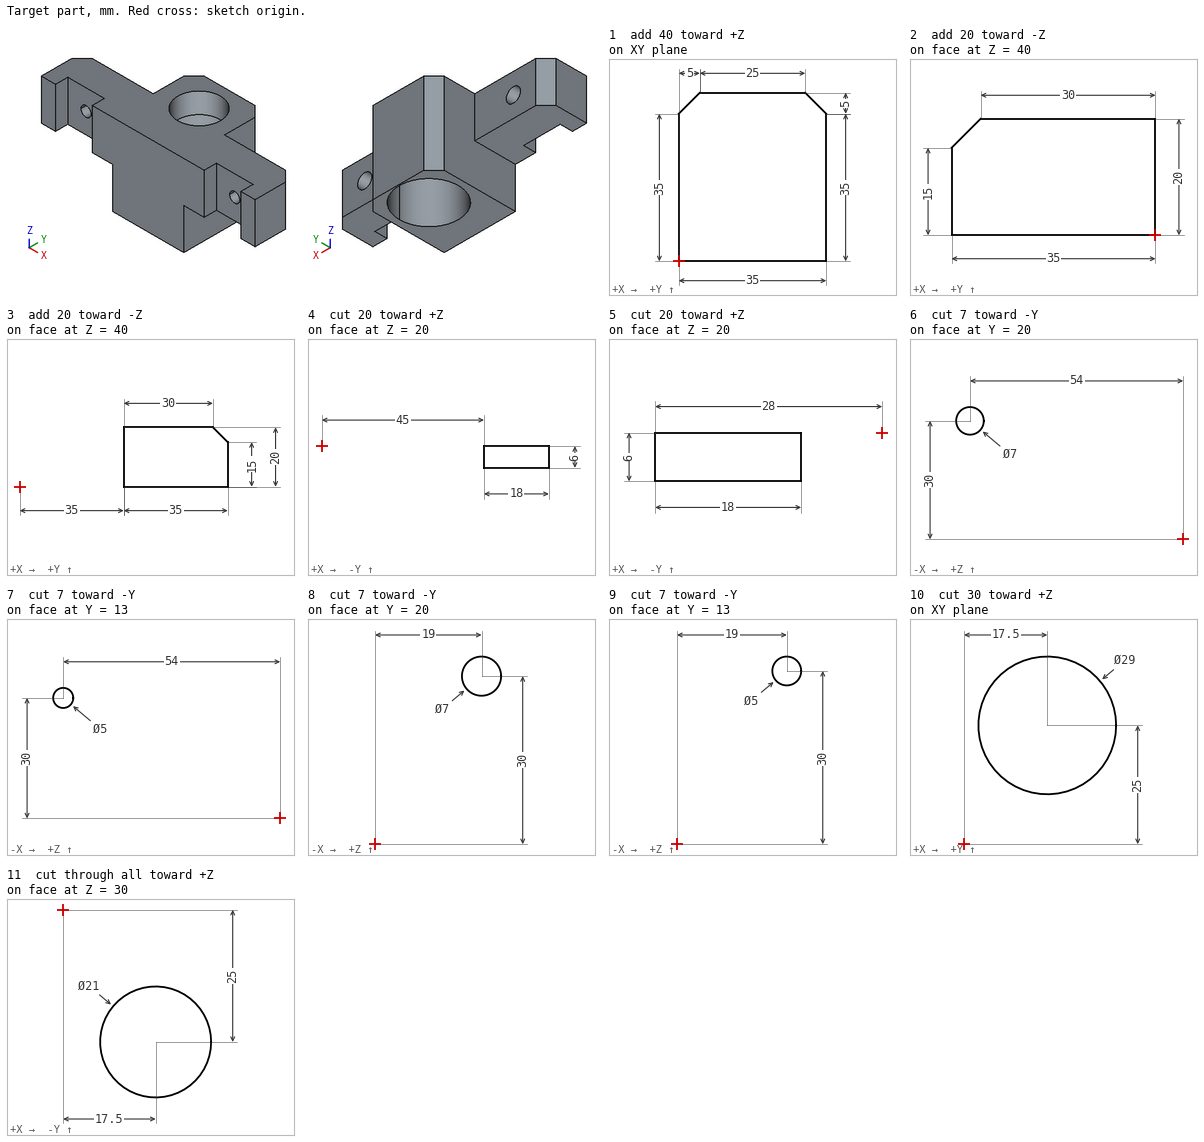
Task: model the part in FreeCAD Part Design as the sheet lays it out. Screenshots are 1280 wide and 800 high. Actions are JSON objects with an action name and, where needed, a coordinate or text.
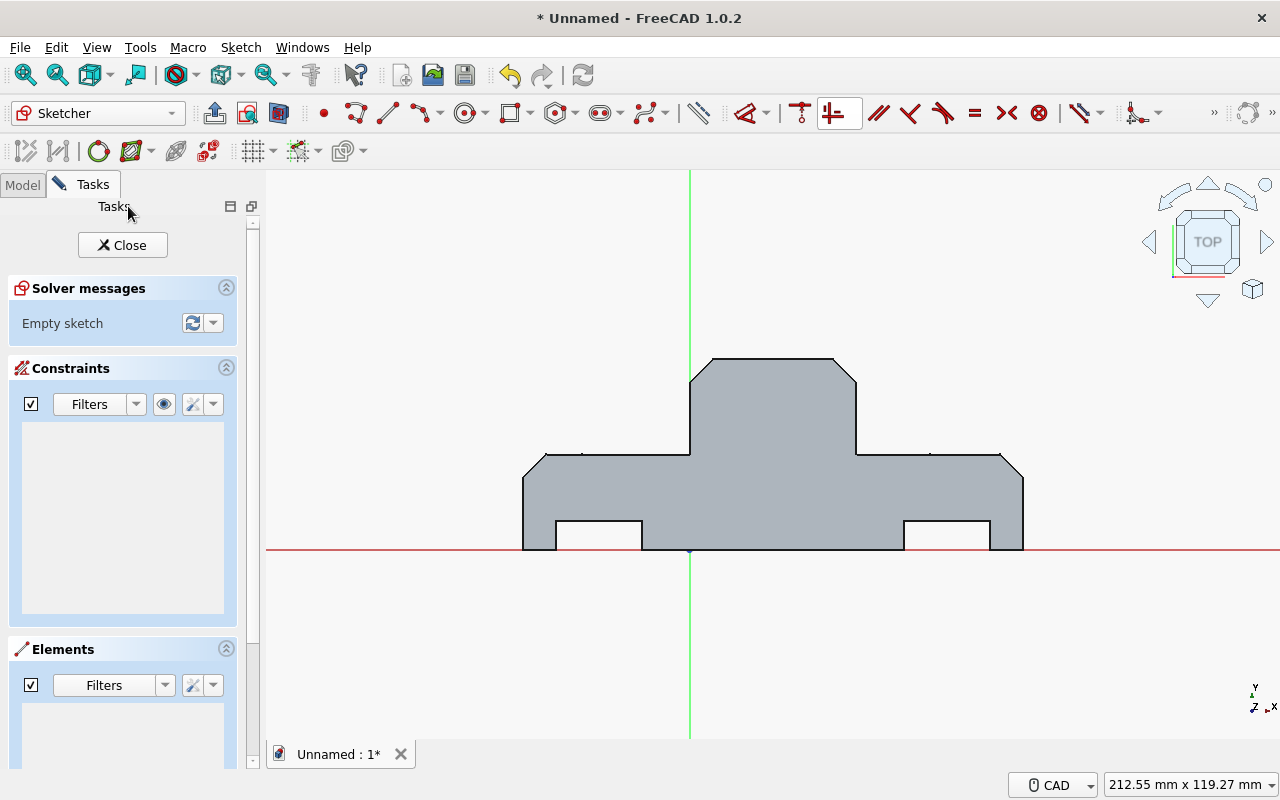
{"action": "left_click", "coordinate": [280, 114]}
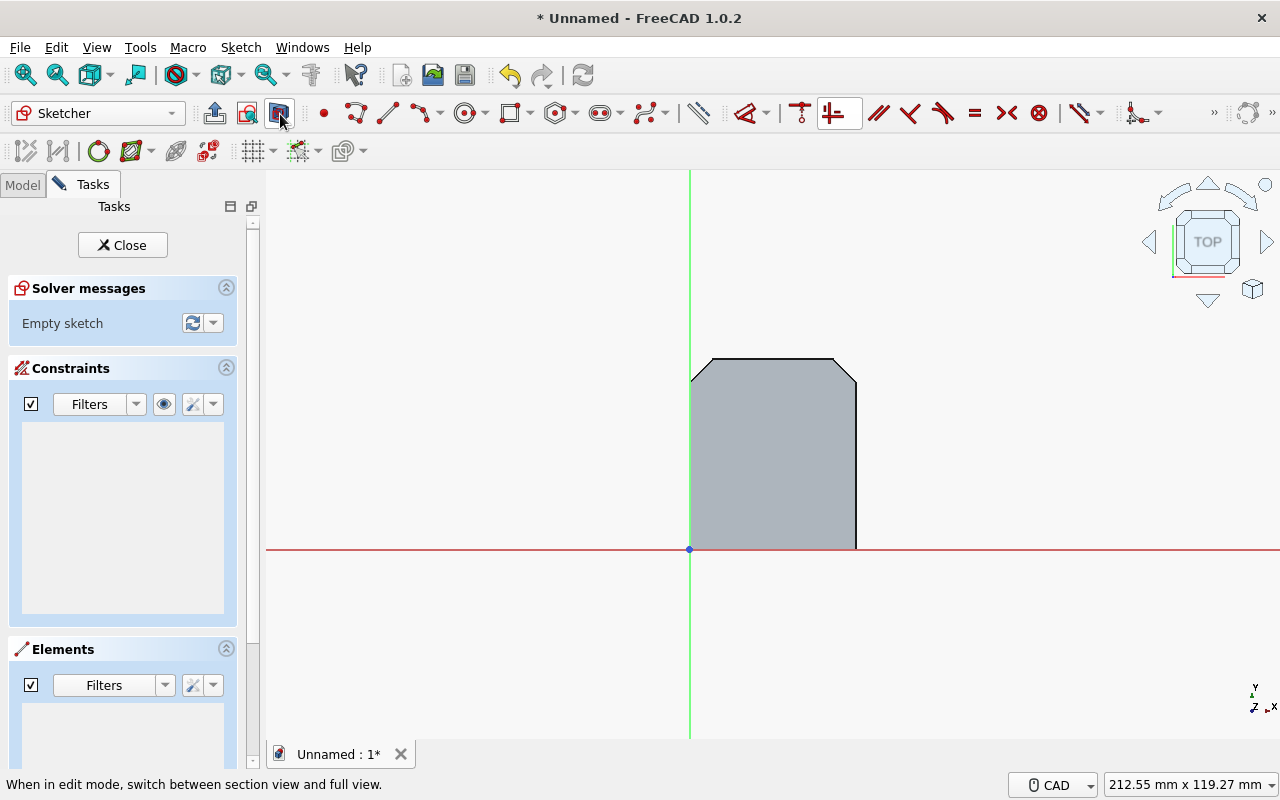
{"action": "scroll", "coordinate": [840, 457], "scroll_direction": "up", "scroll_amount": 3}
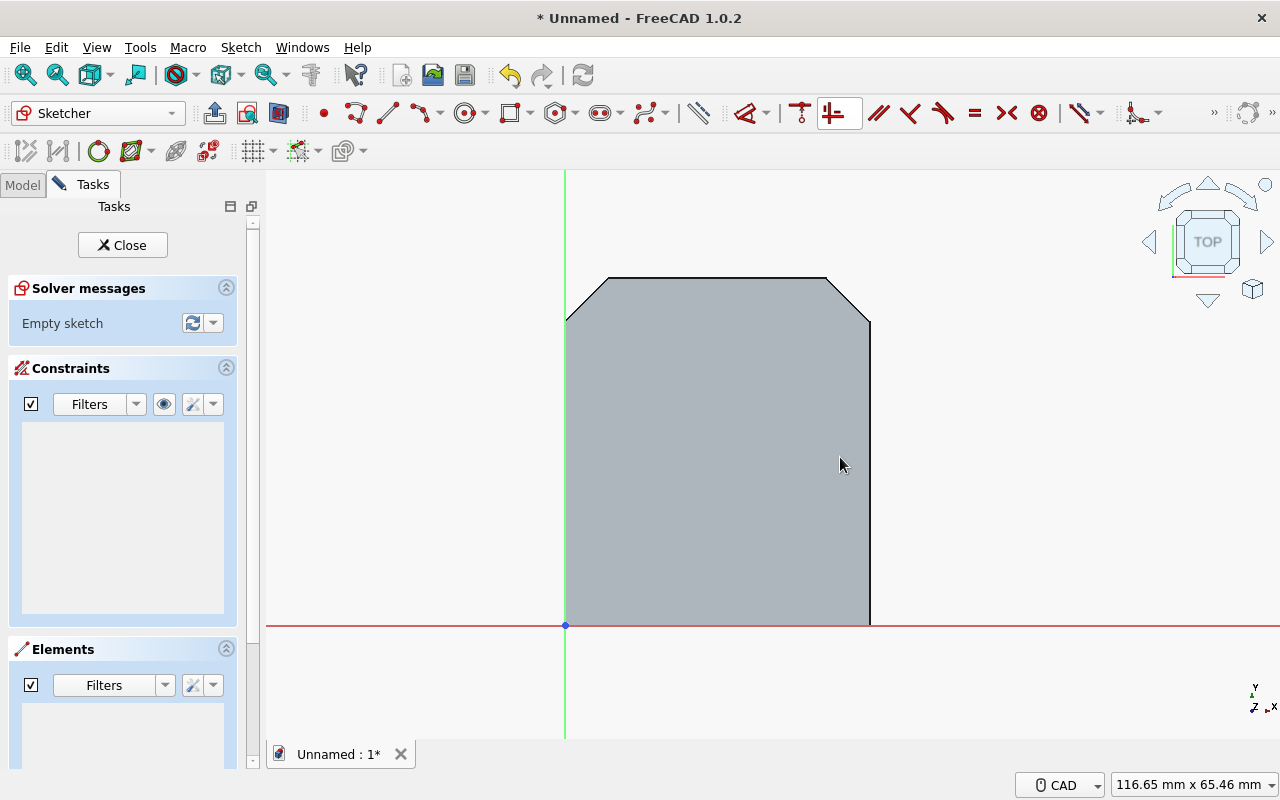
{"action": "left_click", "coordinate": [466, 114]}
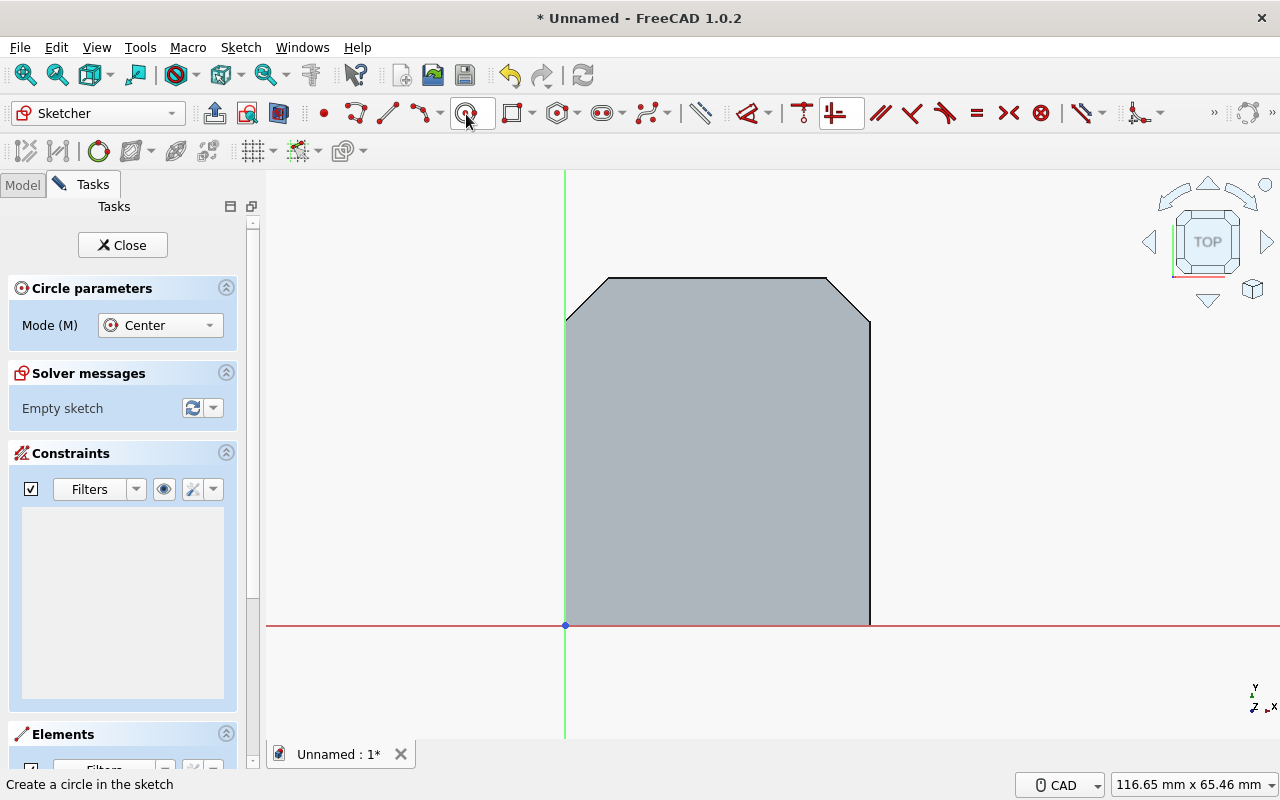
{"action": "left_click", "coordinate": [717, 409]}
{"action": "left_click", "coordinate": [807, 319]}
{"action": "key", "text": "Escape"}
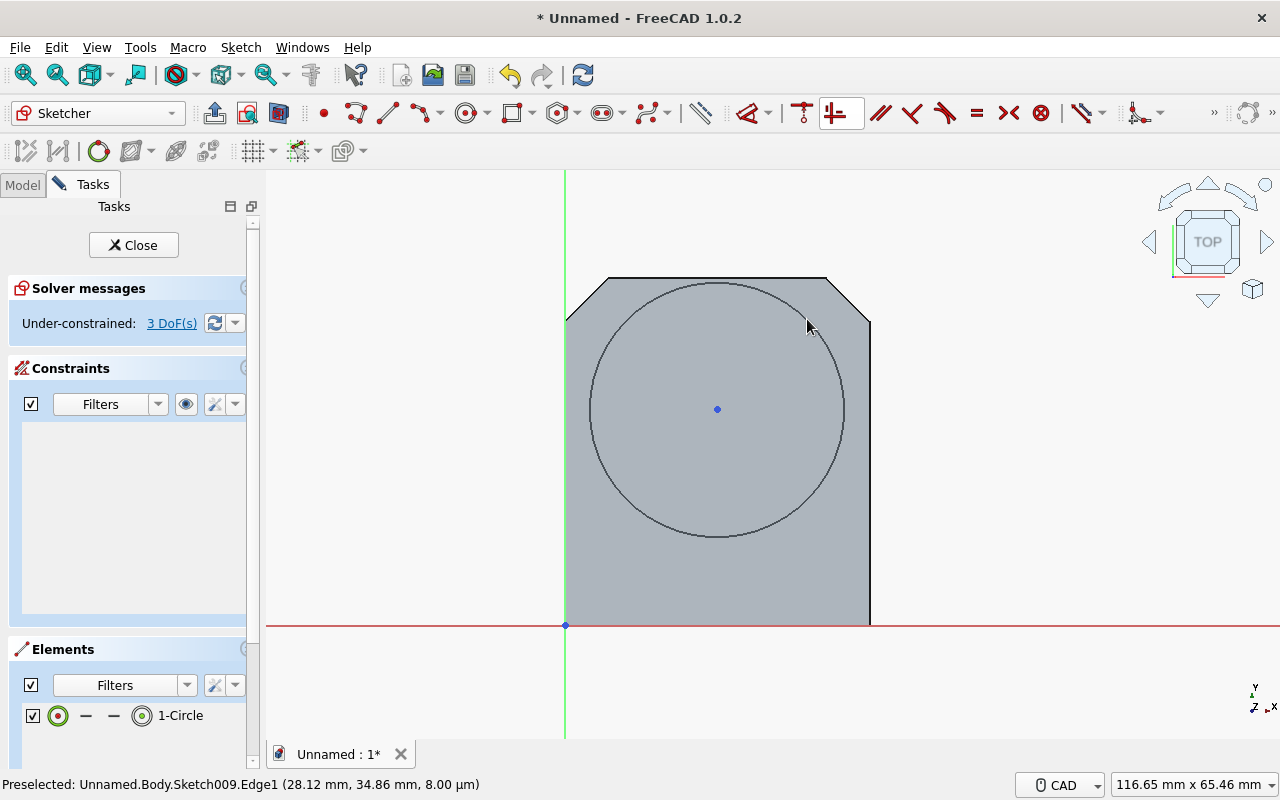
{"action": "left_click", "coordinate": [748, 114]}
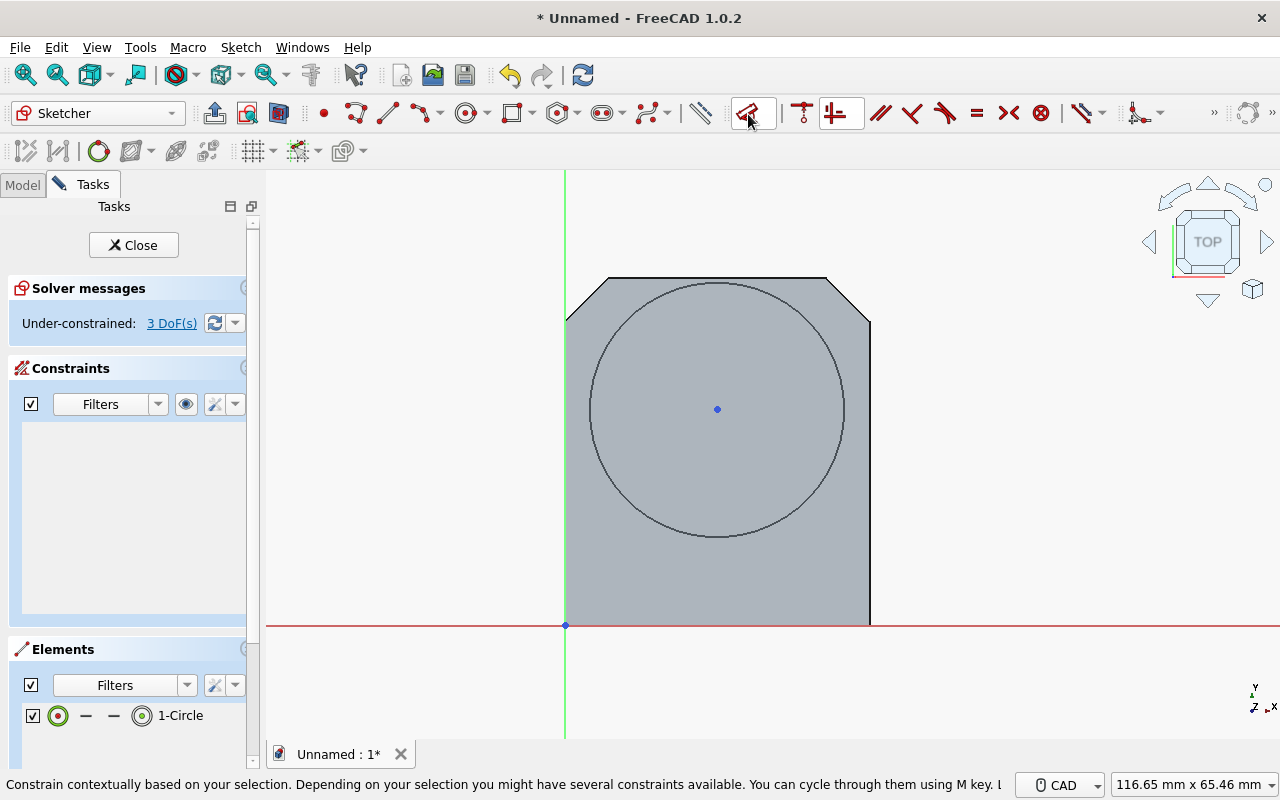
{"action": "left_click", "coordinate": [807, 320]}
{"action": "left_click", "coordinate": [830, 297]}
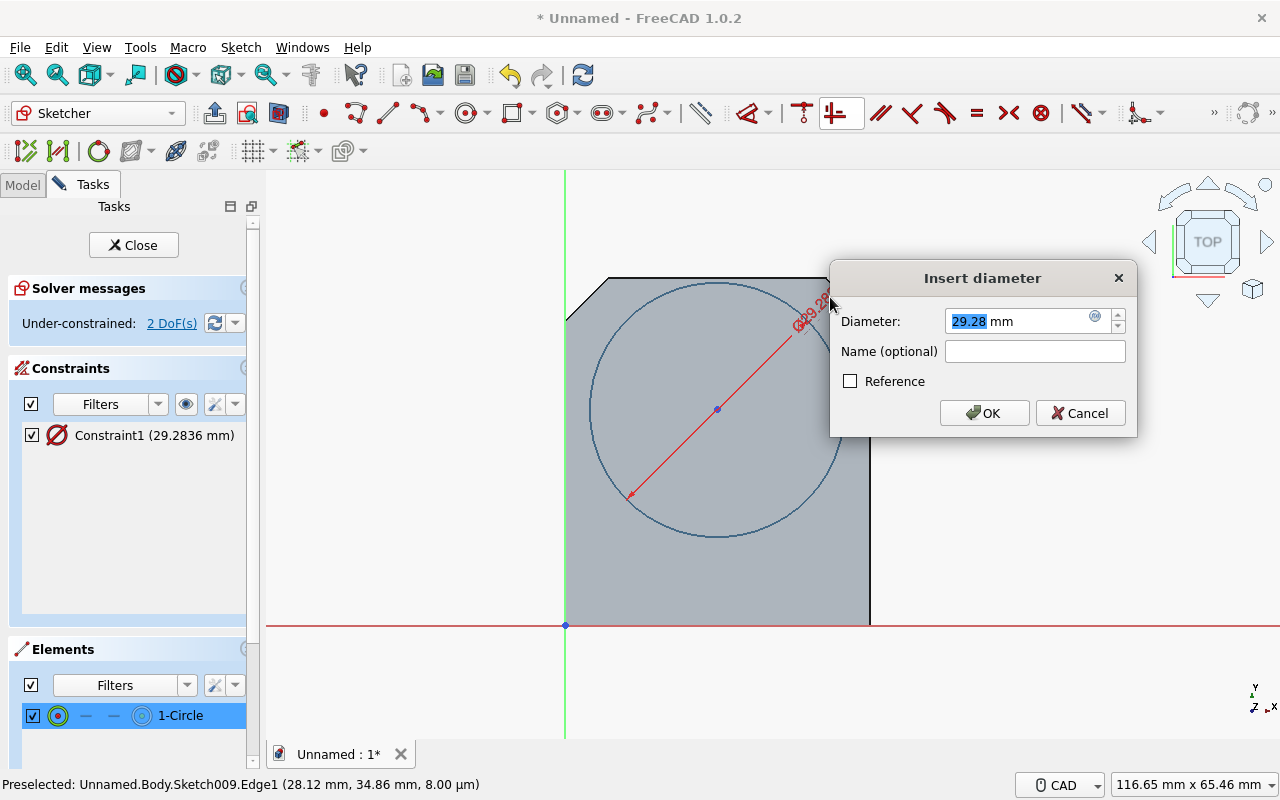
{"action": "type", "text": "29"}
{"action": "key", "text": "Return"}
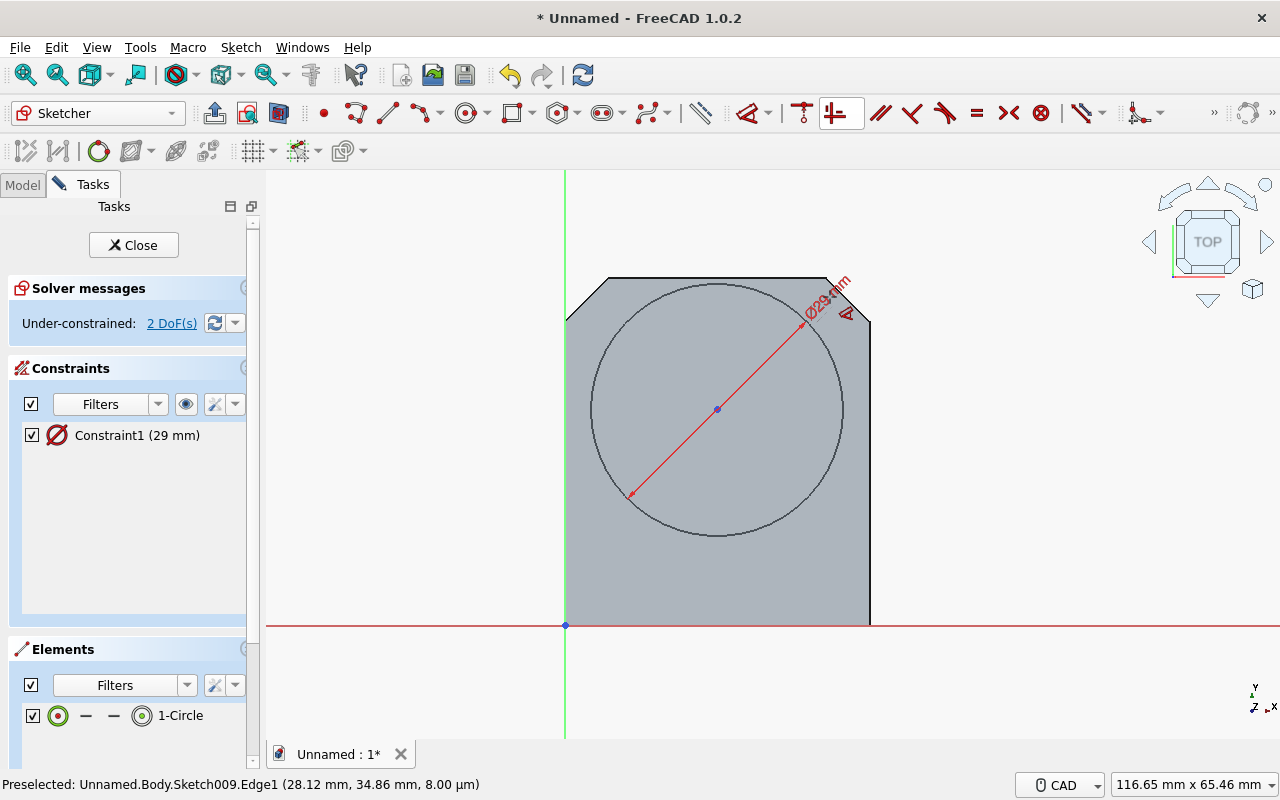
{"action": "left_click", "coordinate": [717, 410]}
{"action": "left_click", "coordinate": [531, 518]}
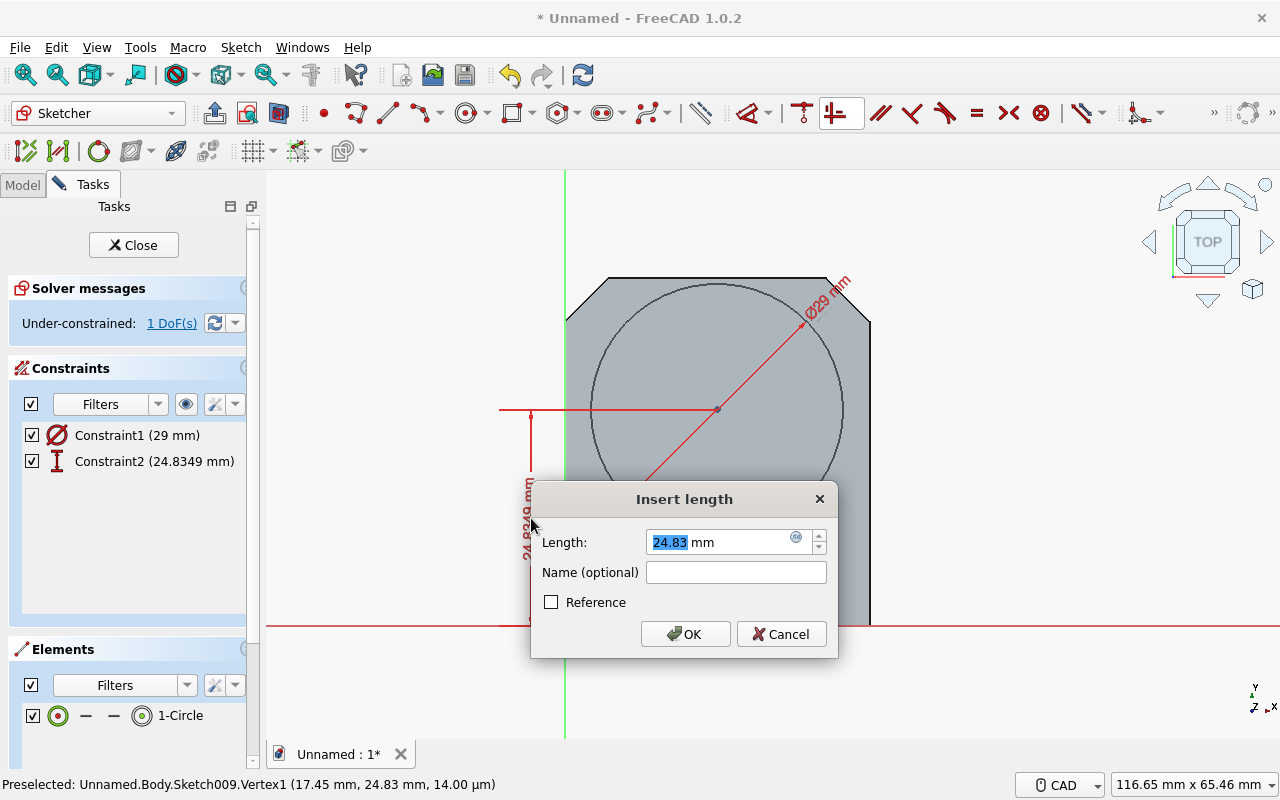
{"action": "type", "text": "25"}
{"action": "key", "text": "Return"}